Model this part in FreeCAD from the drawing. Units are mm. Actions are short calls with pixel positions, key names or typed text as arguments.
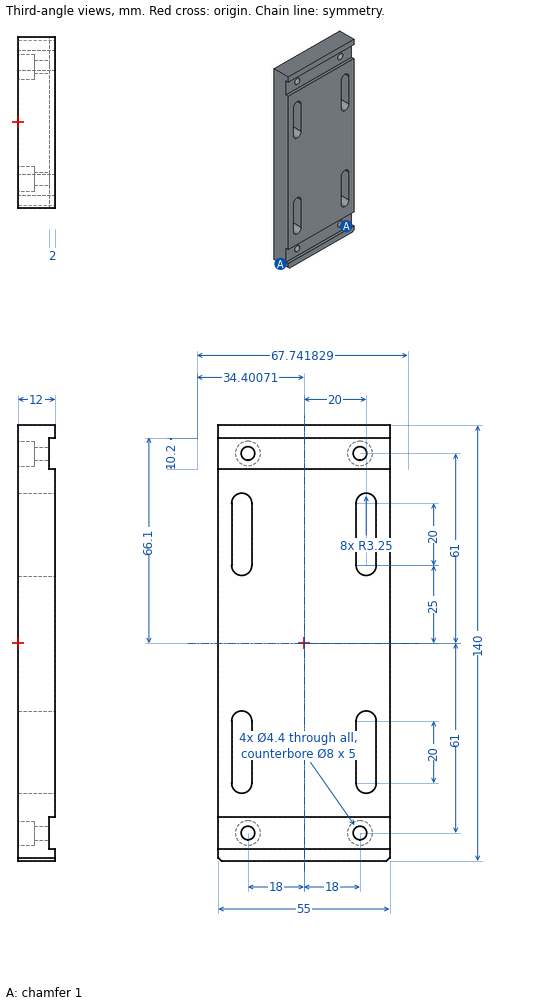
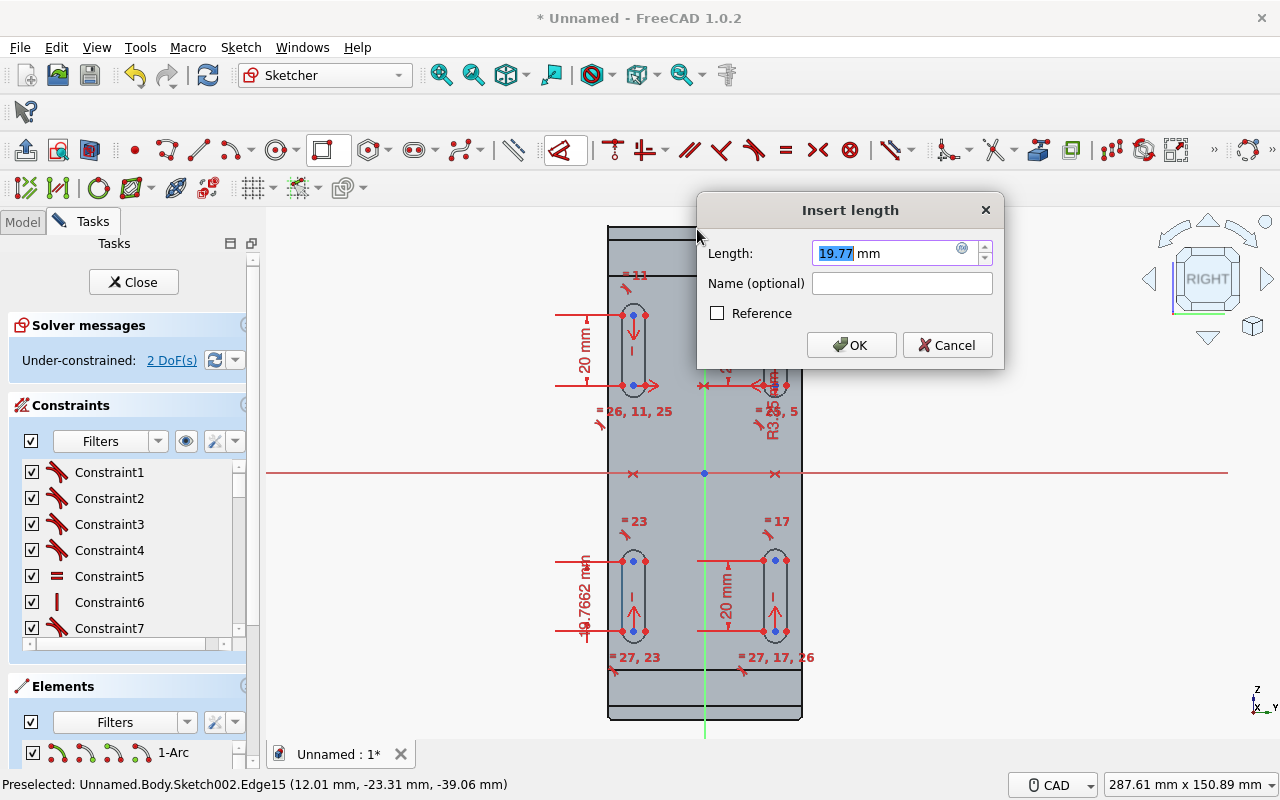
text(20)
key(Return)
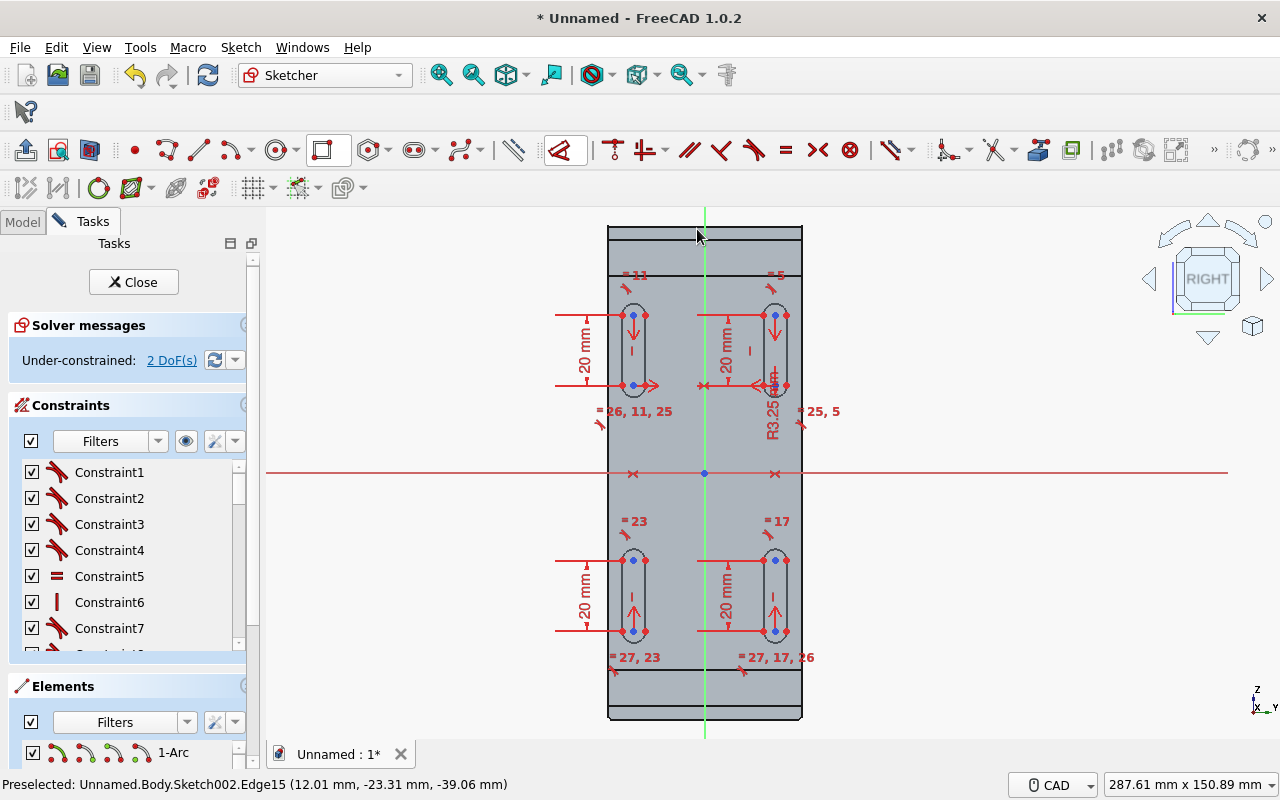
click(764, 386)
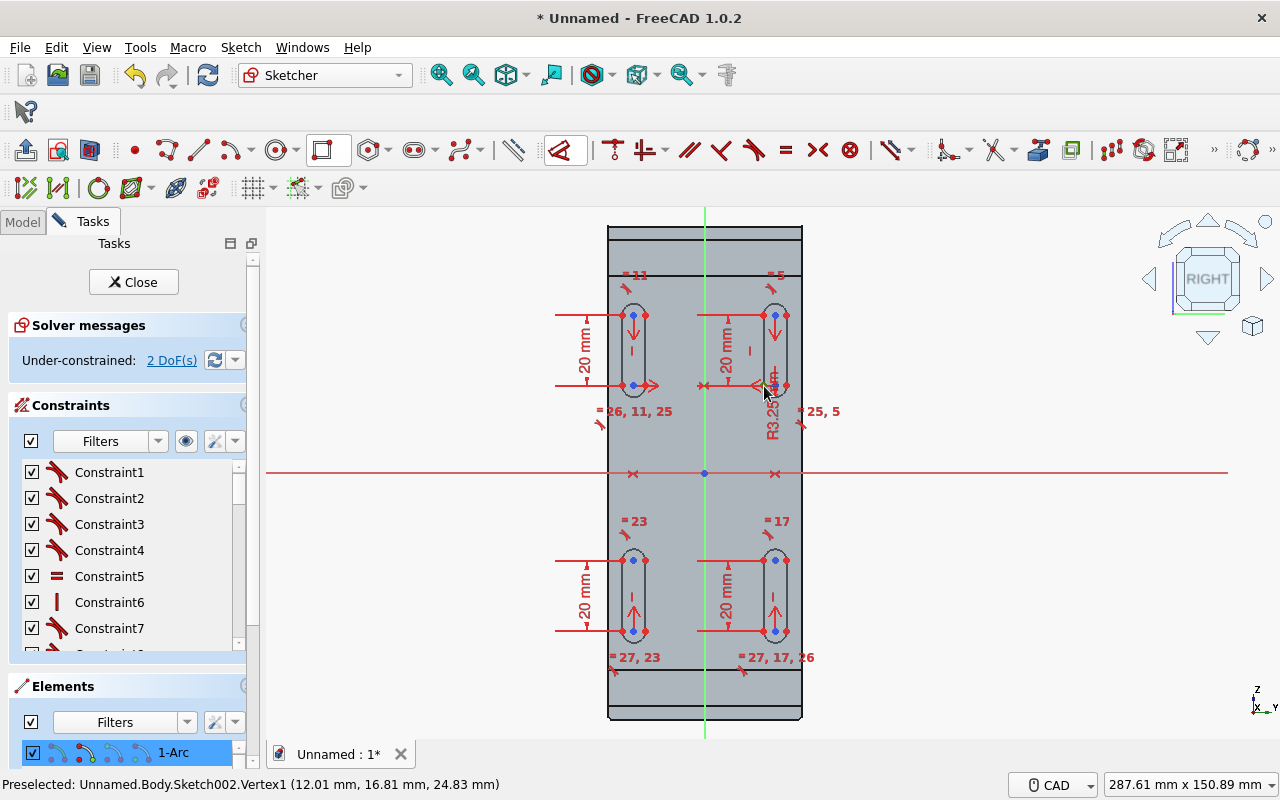
click(582, 150)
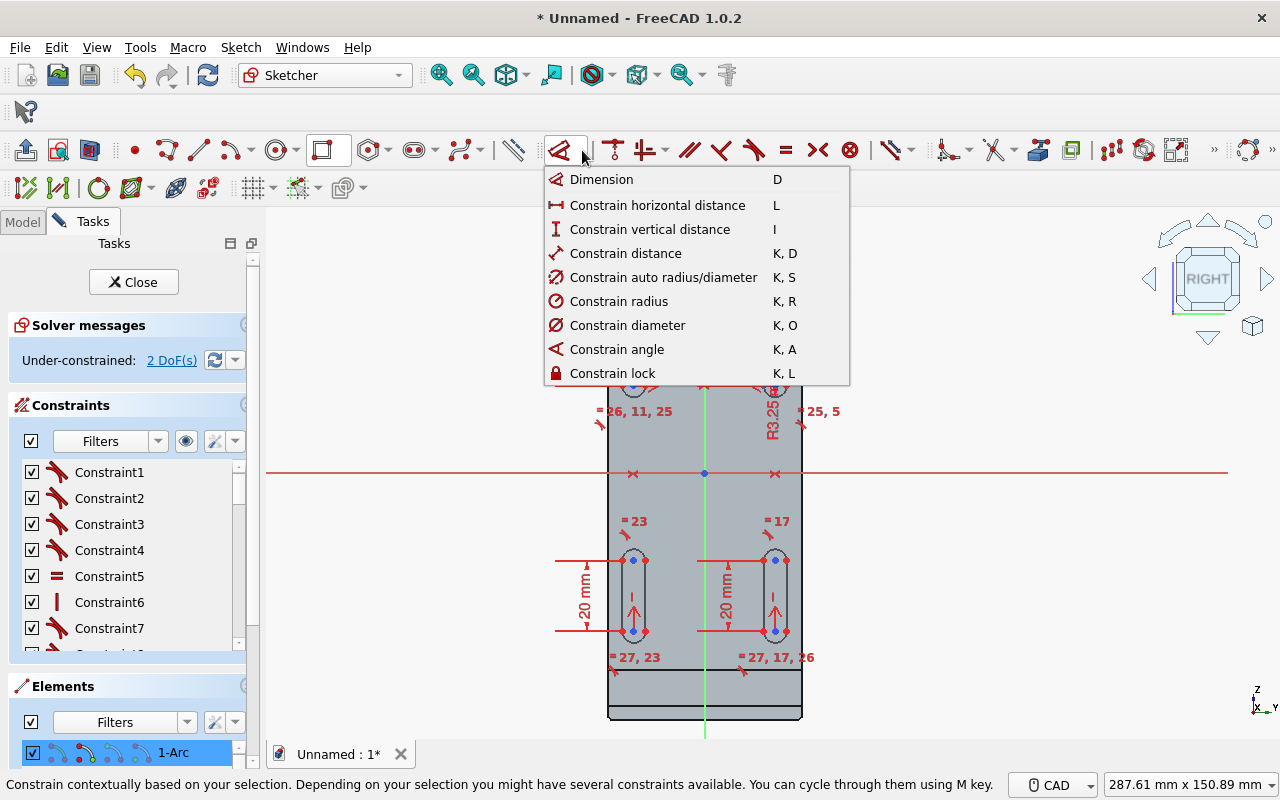
click(697, 229)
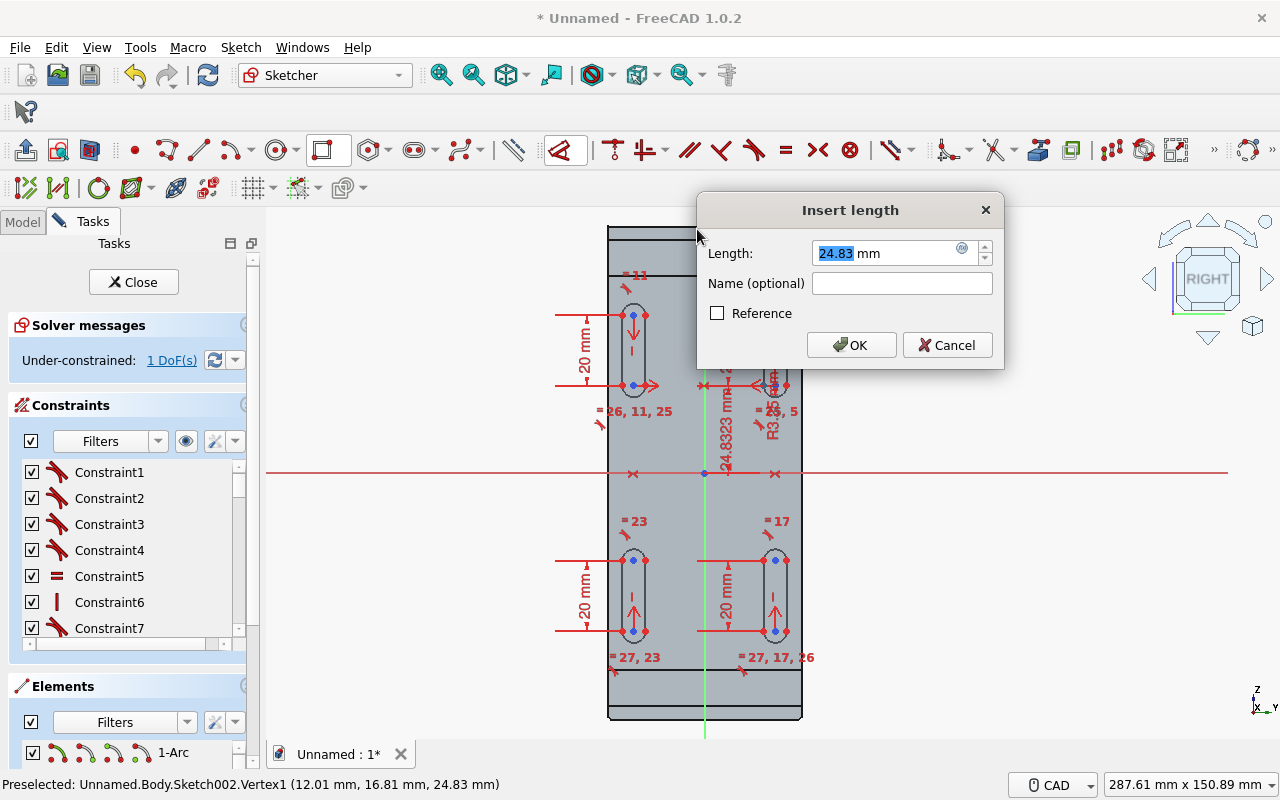
text(25)
key(Return)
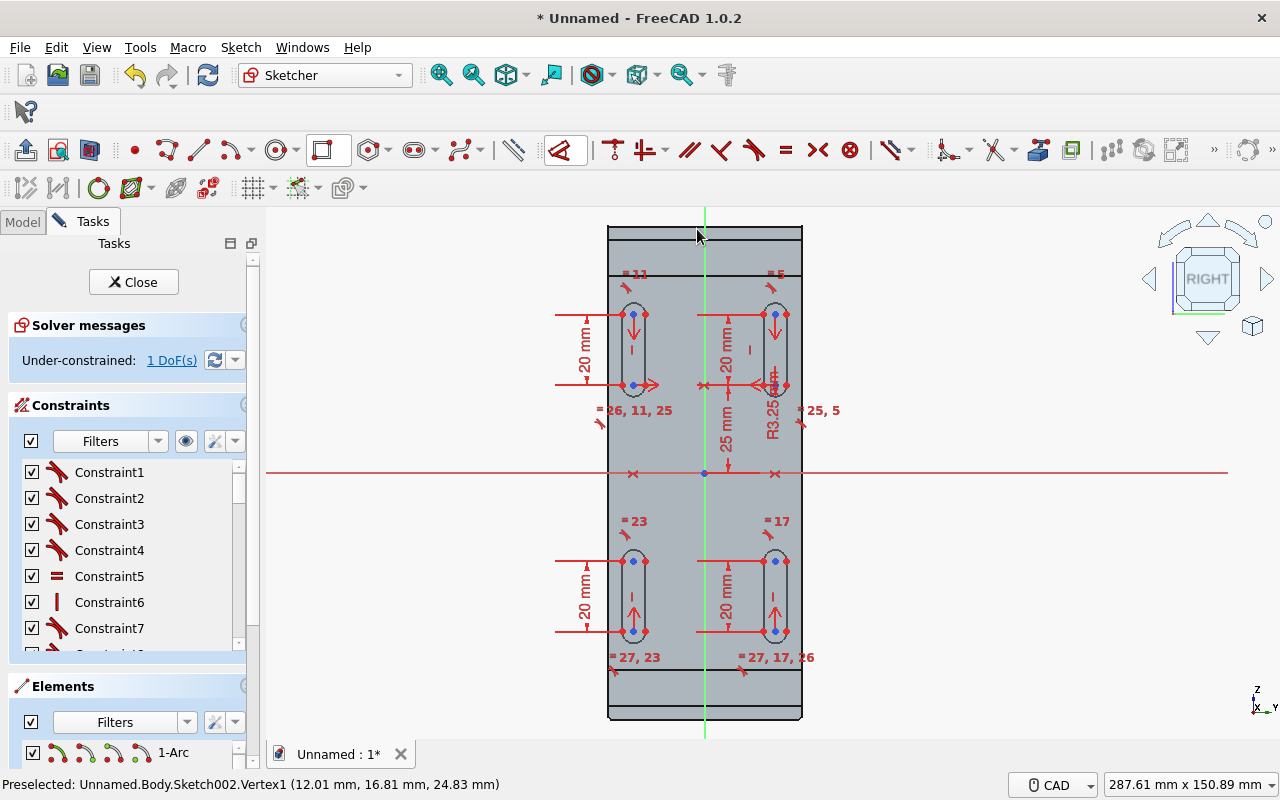
click(775, 385)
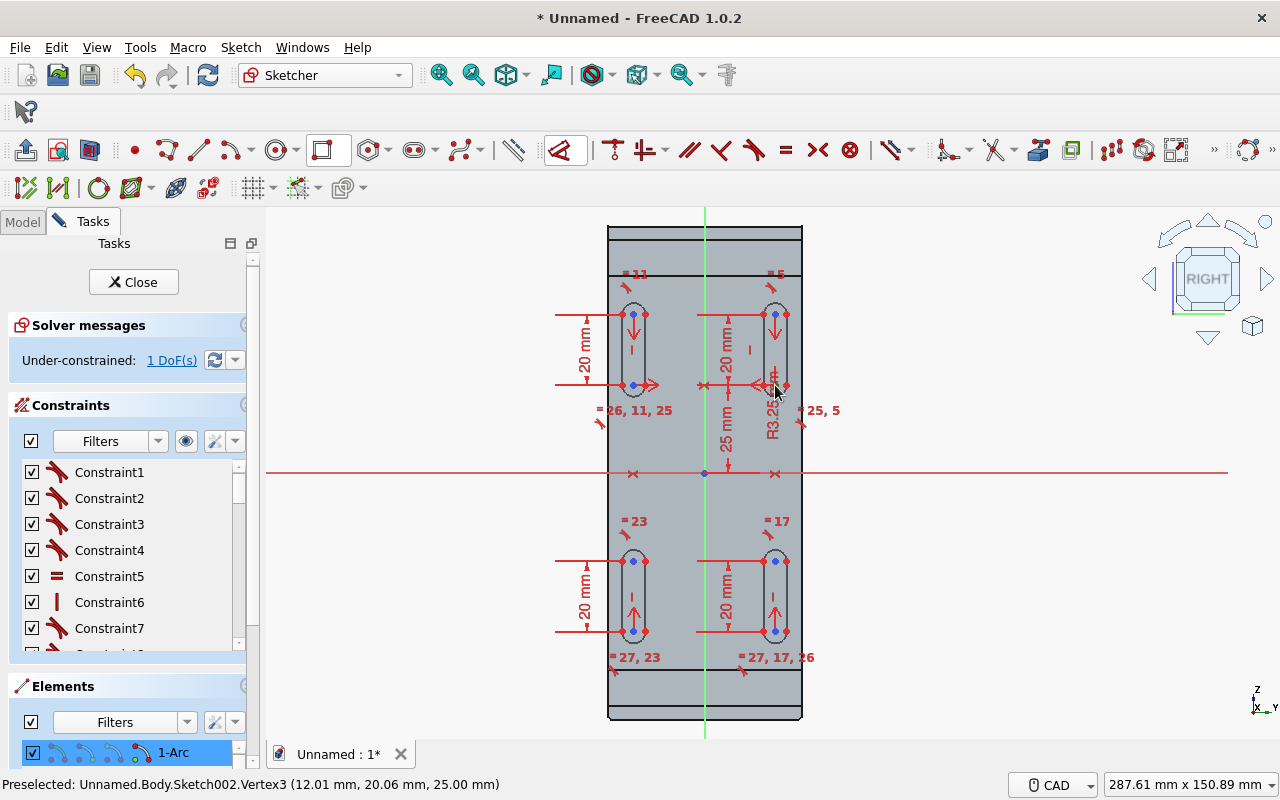
click(582, 150)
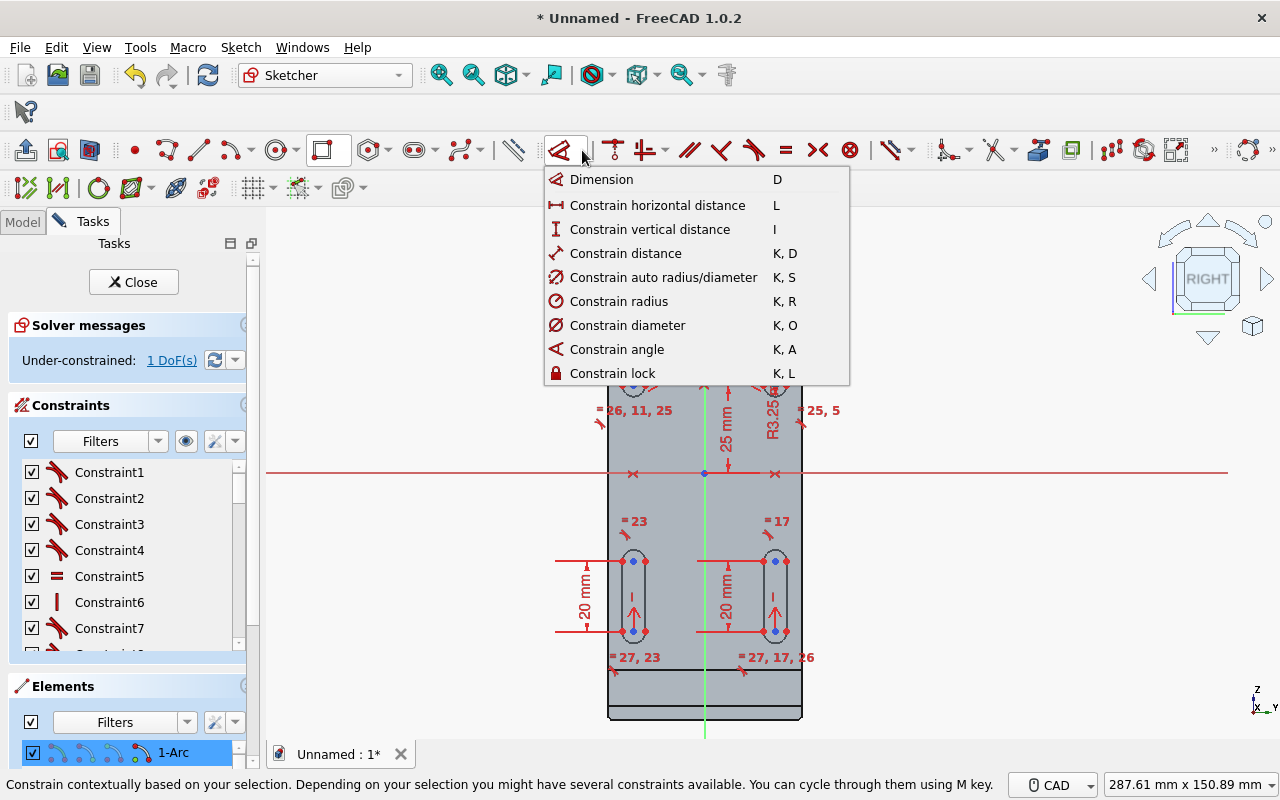
click(697, 205)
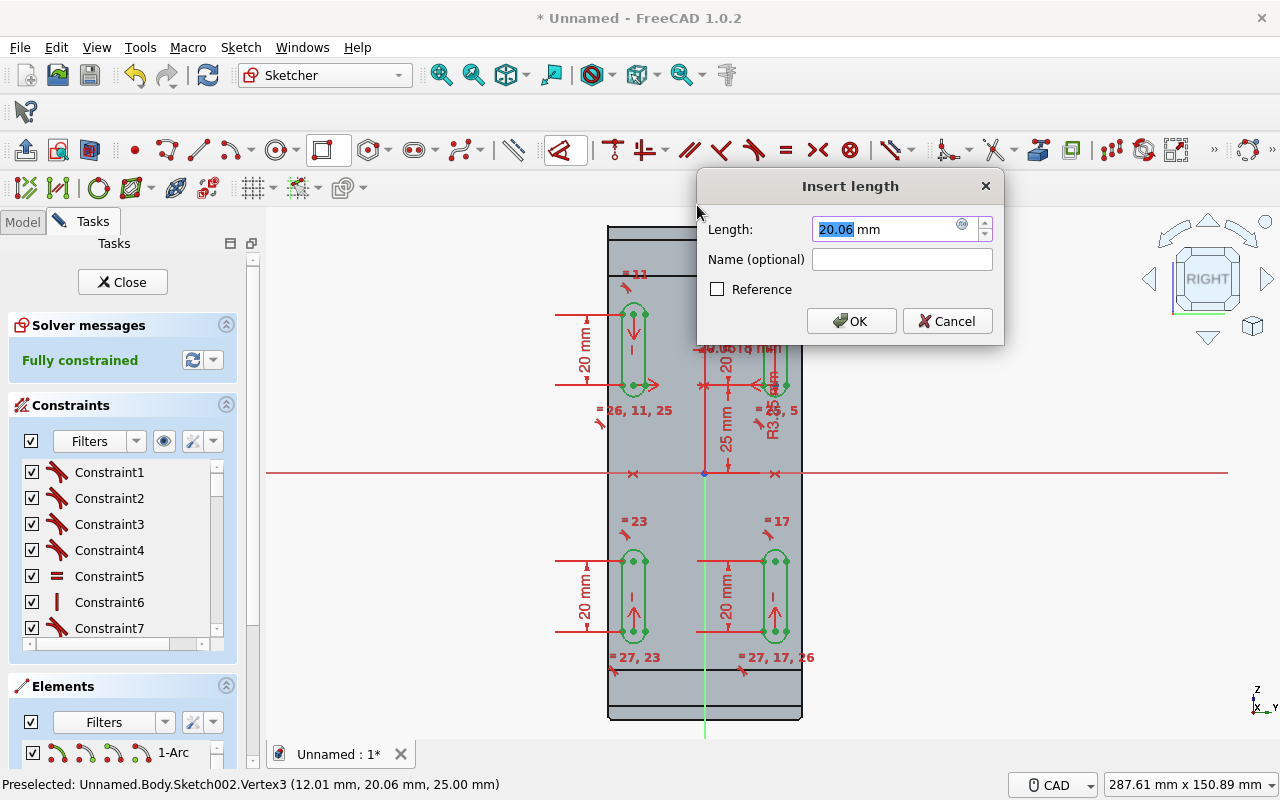
text(20)
key(Return)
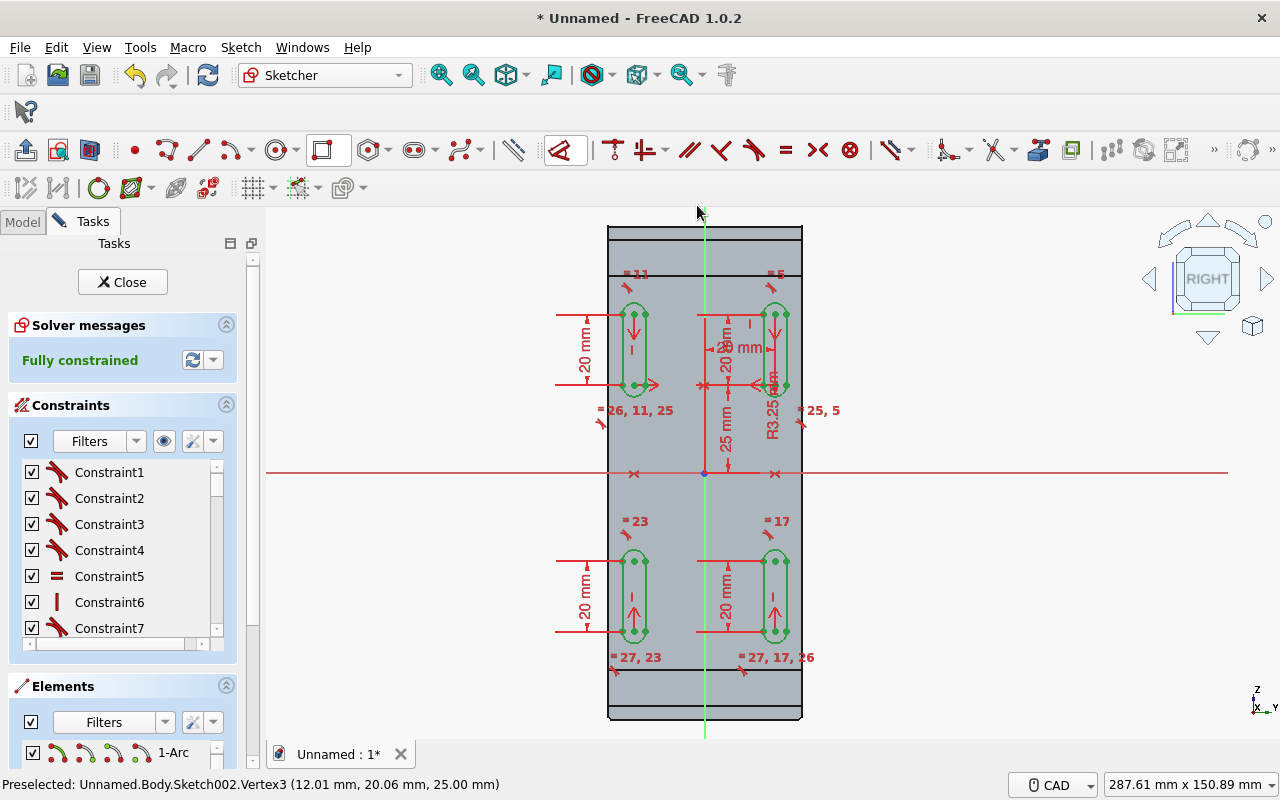
click(123, 282)